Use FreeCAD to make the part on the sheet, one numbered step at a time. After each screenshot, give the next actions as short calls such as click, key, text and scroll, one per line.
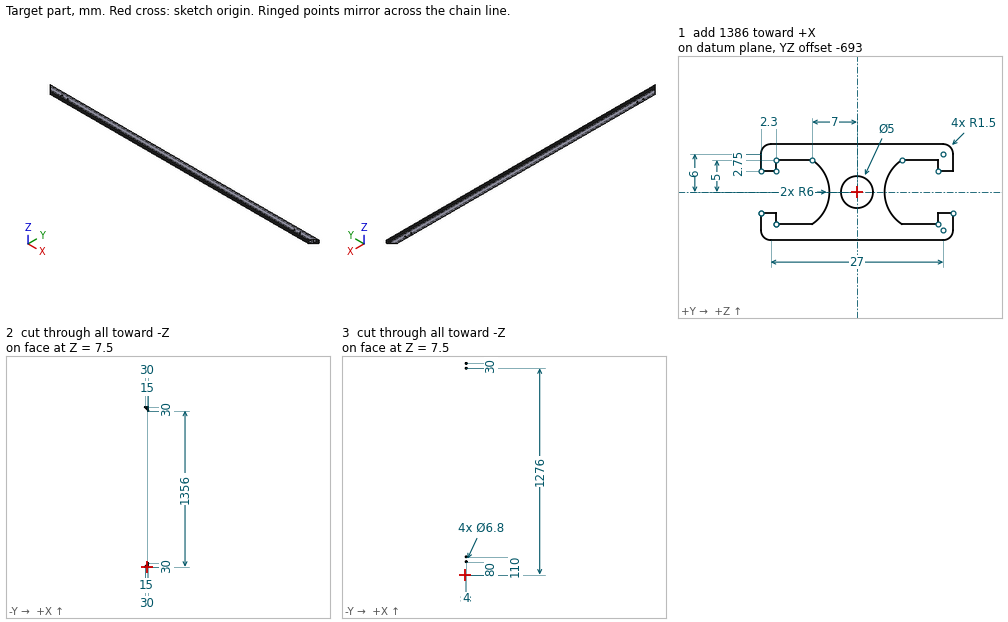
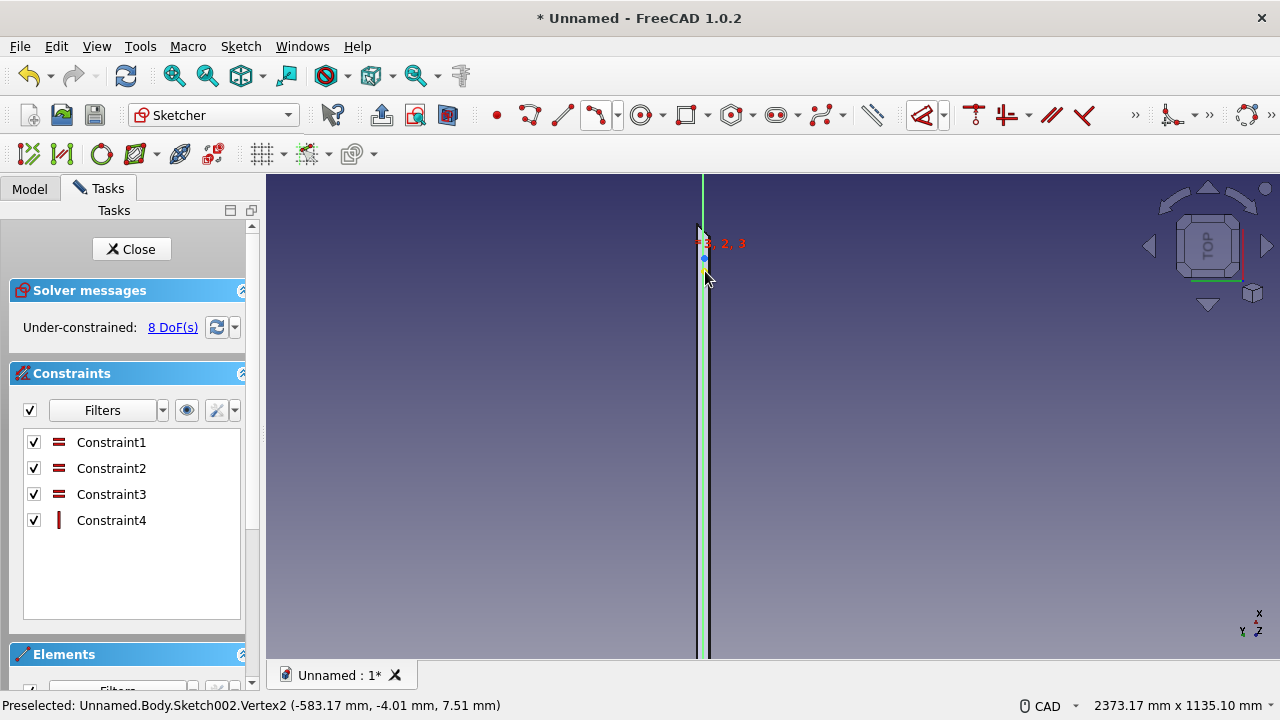
click(705, 271)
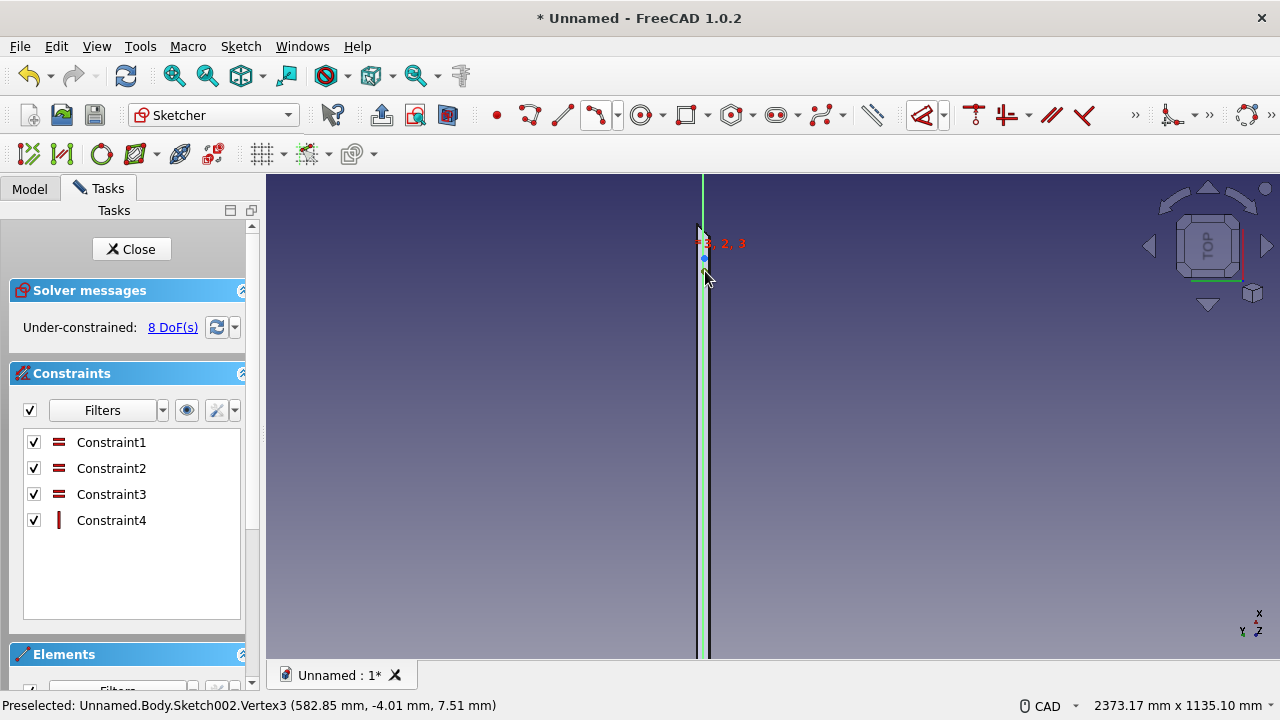
key(v)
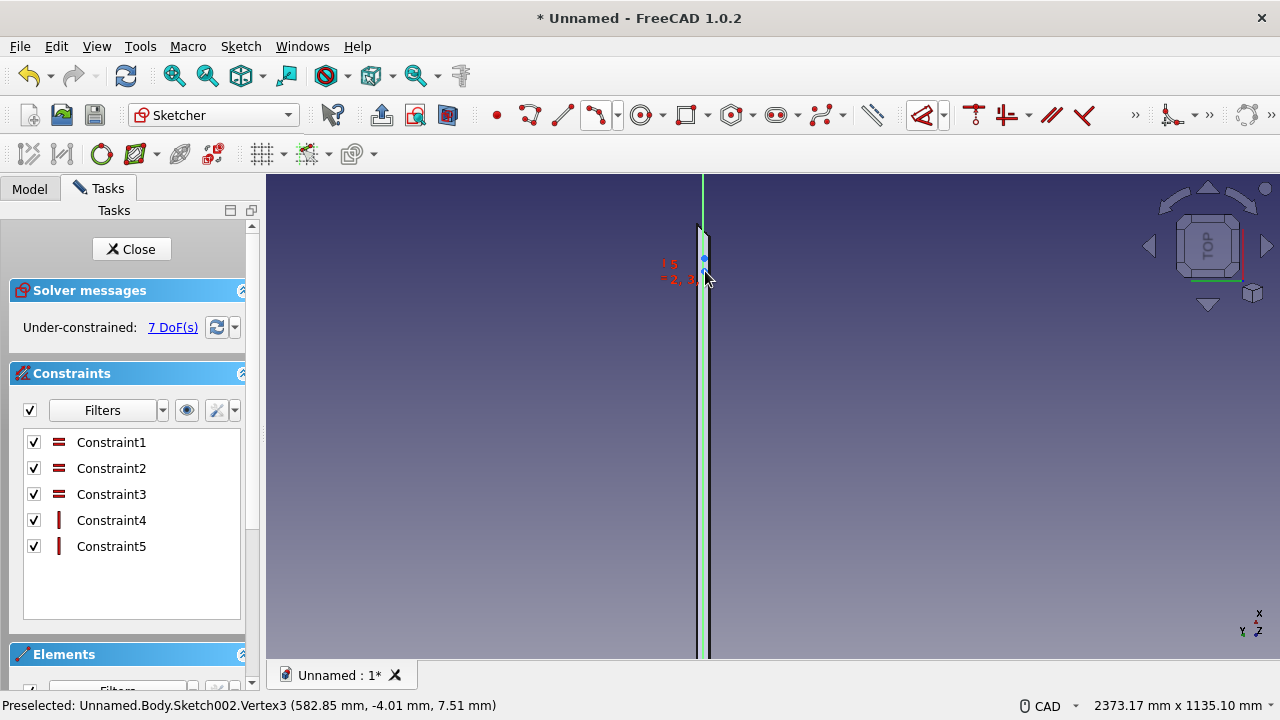
scroll(705, 271, up, 4)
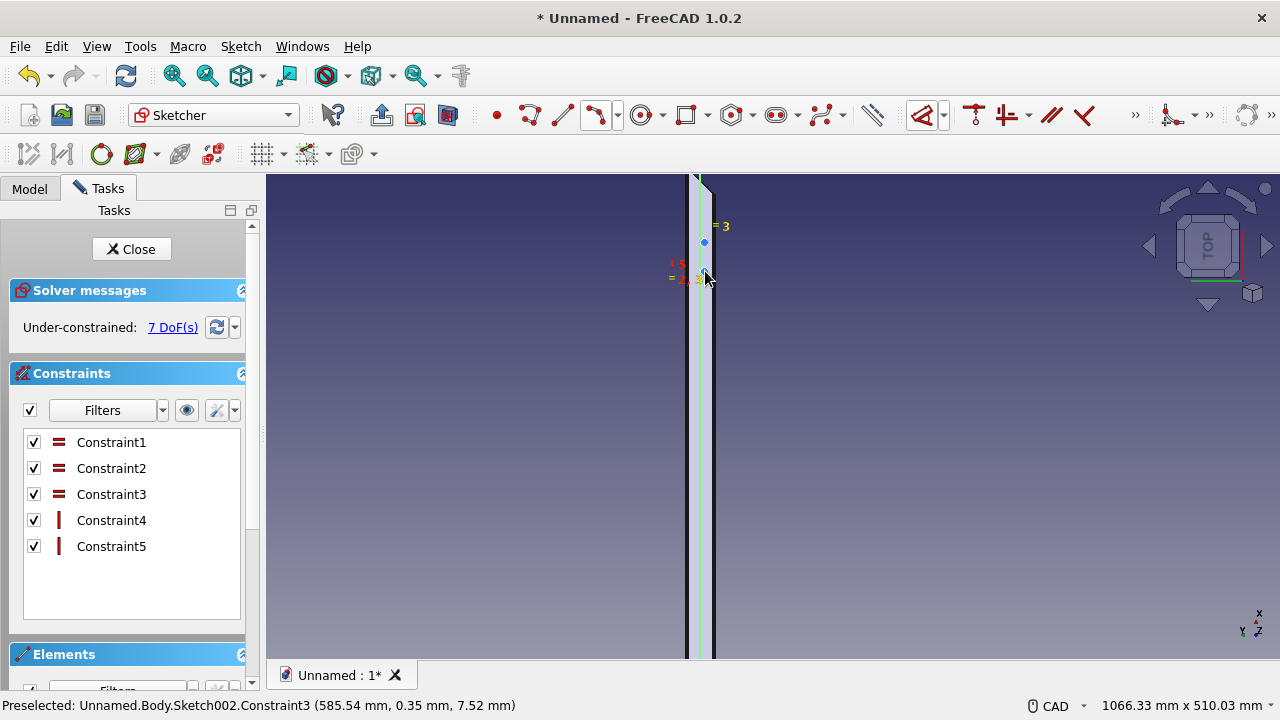
click(704, 271)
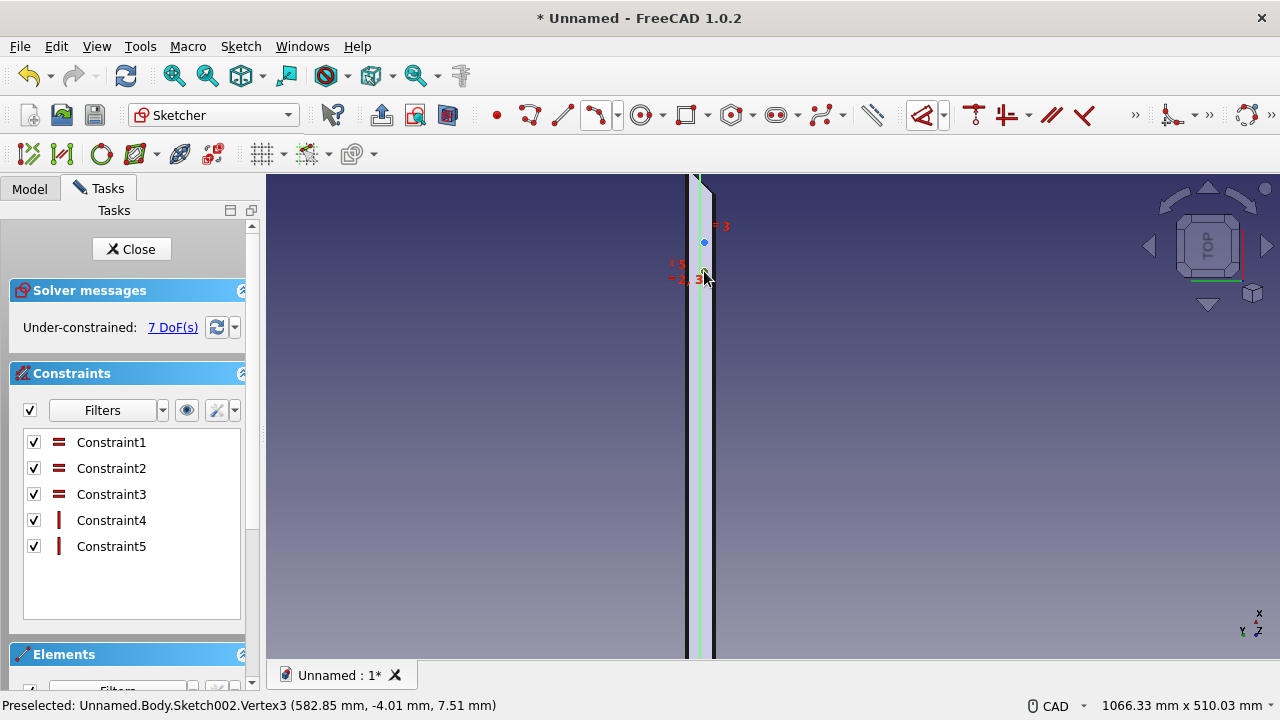
click(704, 242)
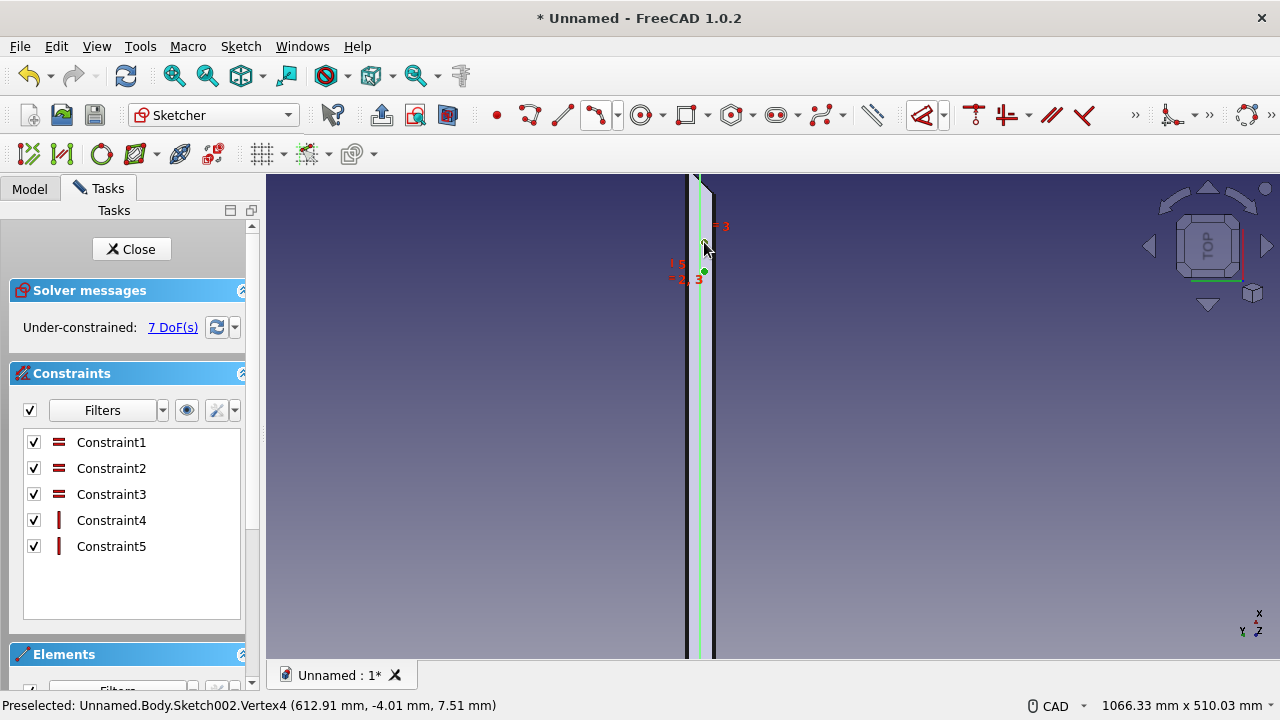
click(1028, 116)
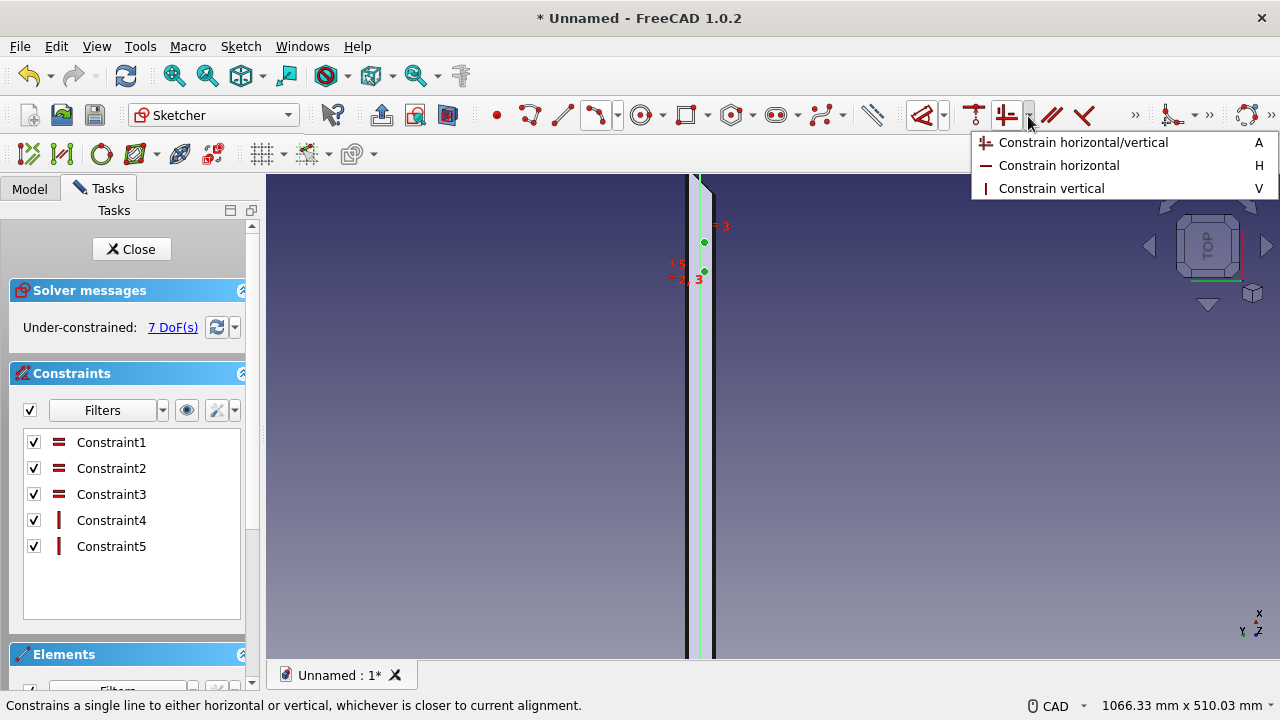
click(1125, 188)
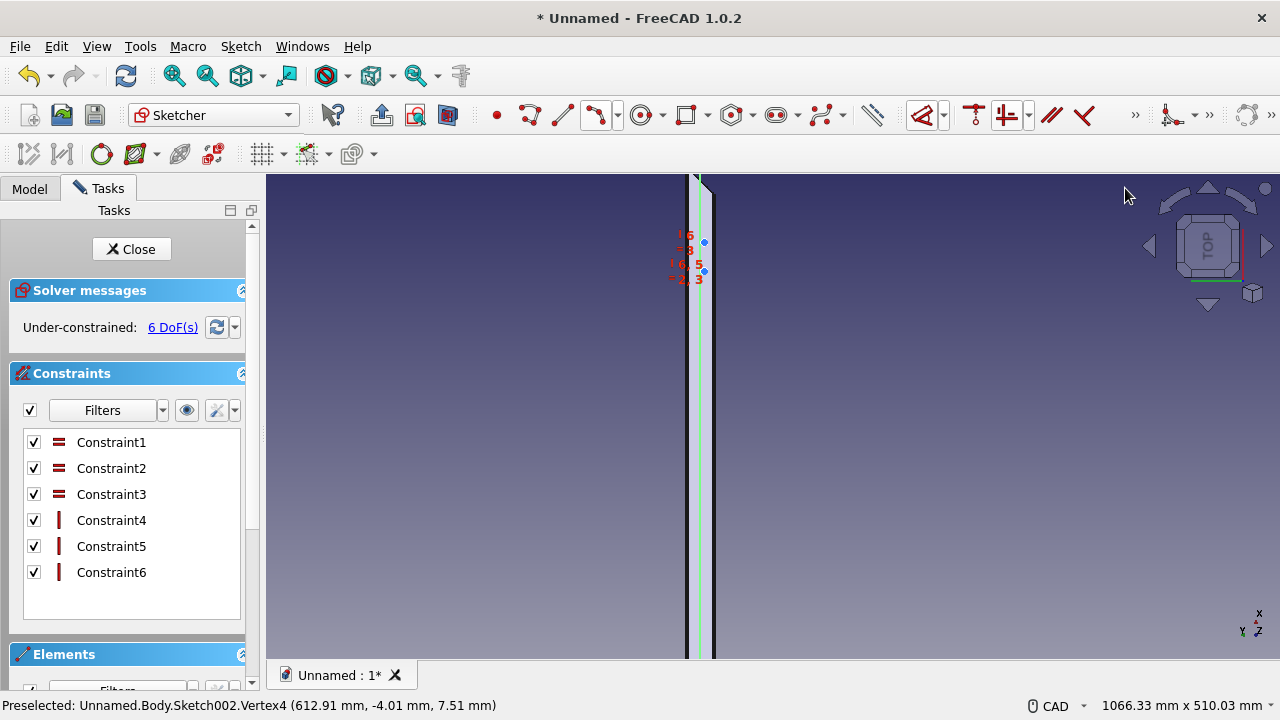
scroll(705, 271, down, 7)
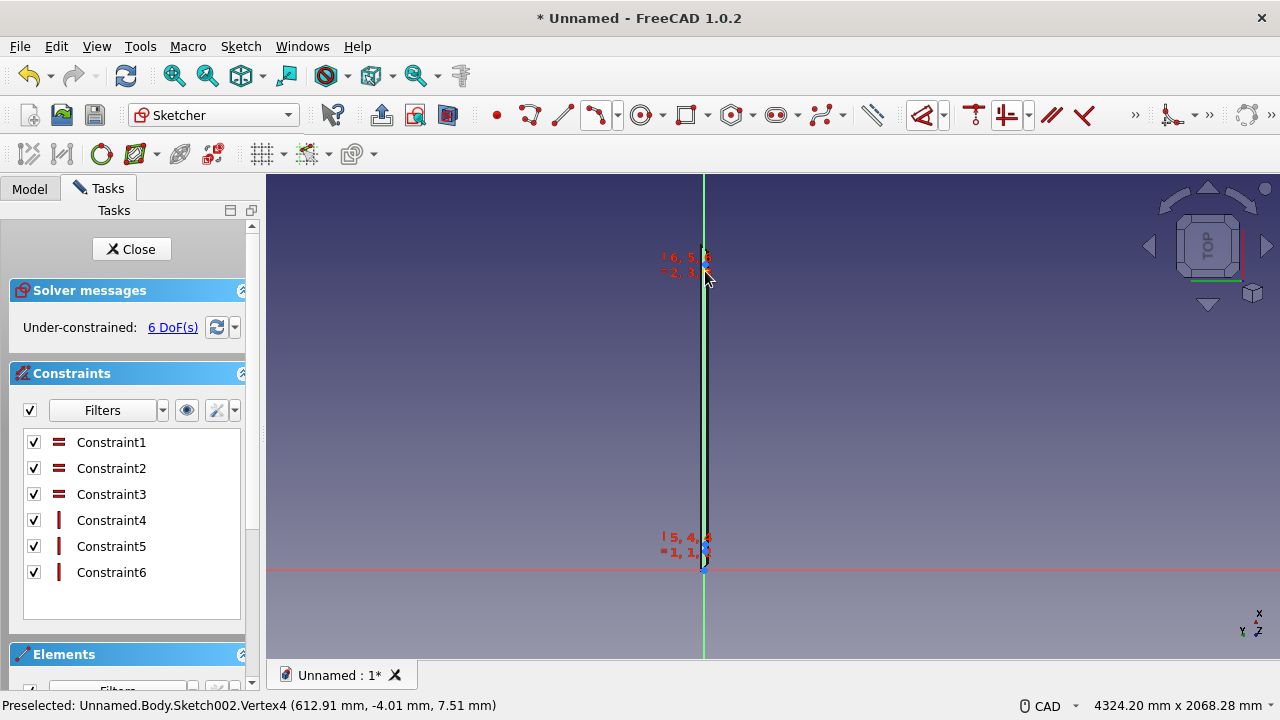
scroll(705, 551, up, 17)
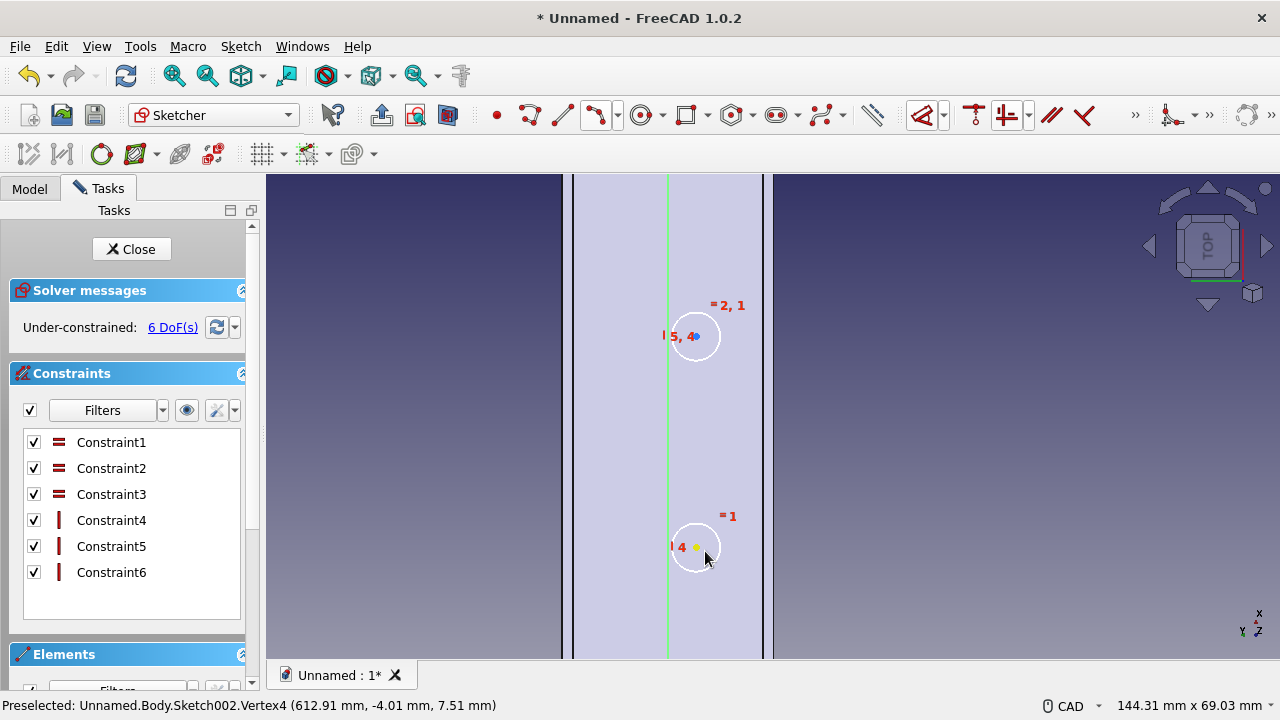
click(697, 524)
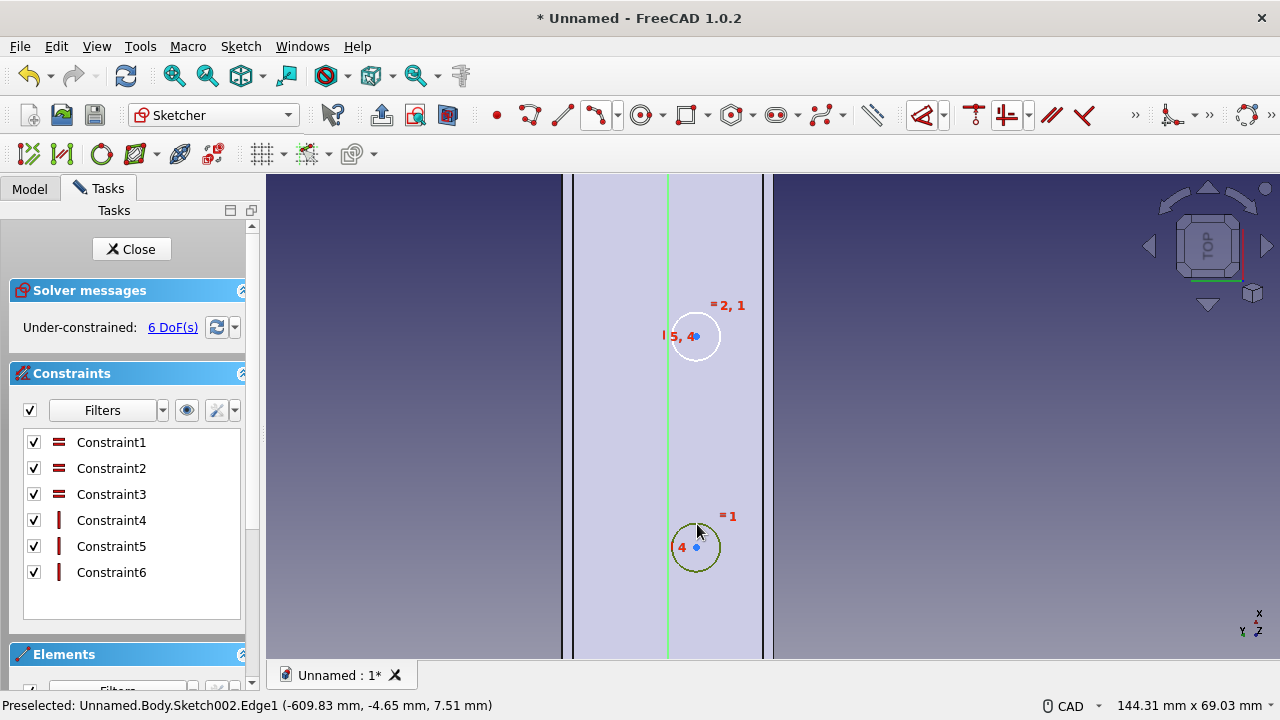
key(k)
key(o)